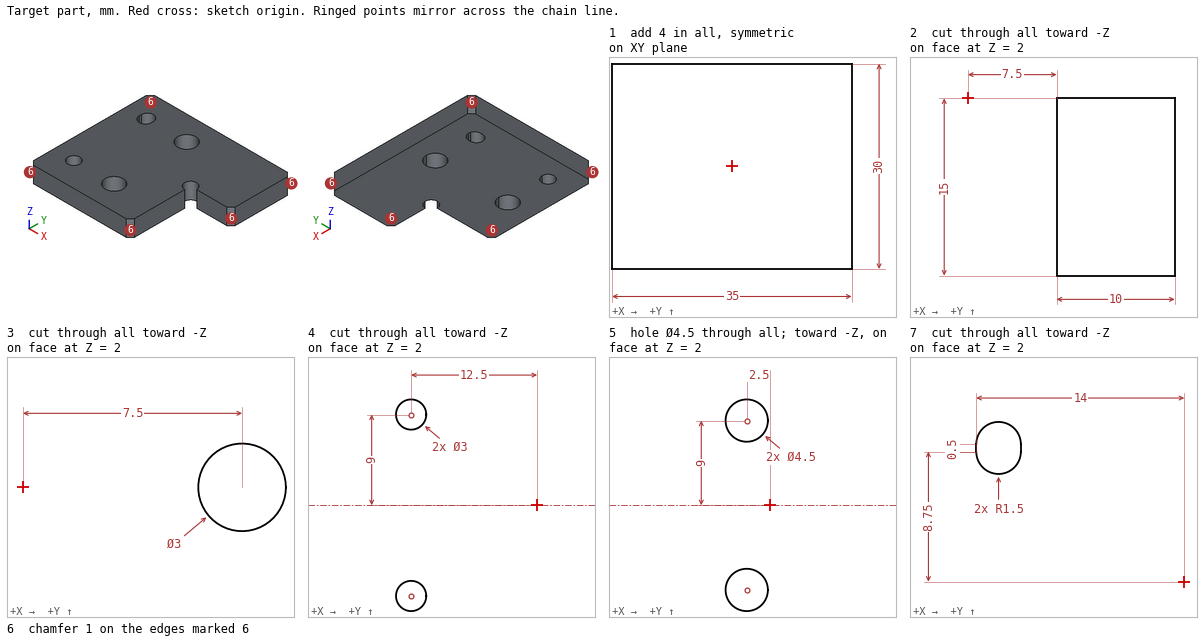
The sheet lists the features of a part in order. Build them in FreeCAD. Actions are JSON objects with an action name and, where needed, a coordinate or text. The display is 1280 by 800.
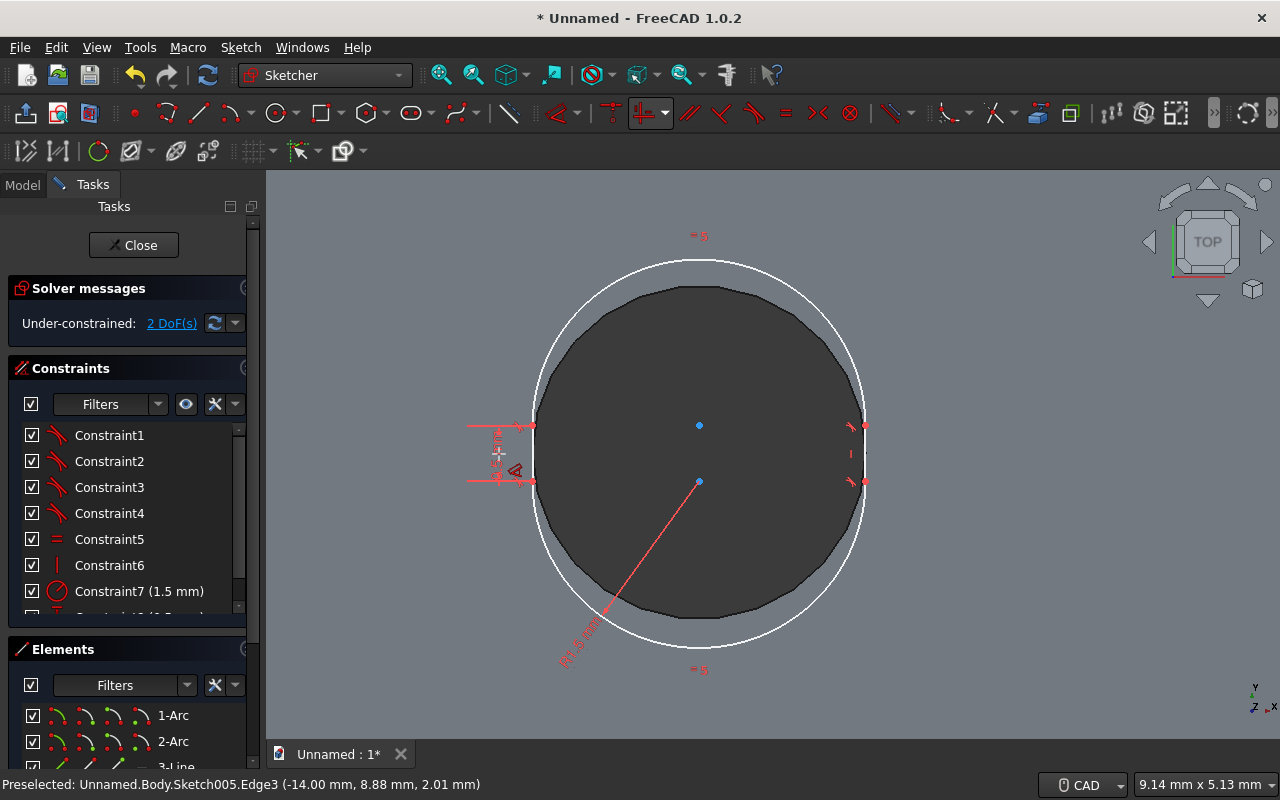
{"action": "left_click", "coordinate": [533, 481]}
{"action": "left_click", "coordinate": [824, 447]}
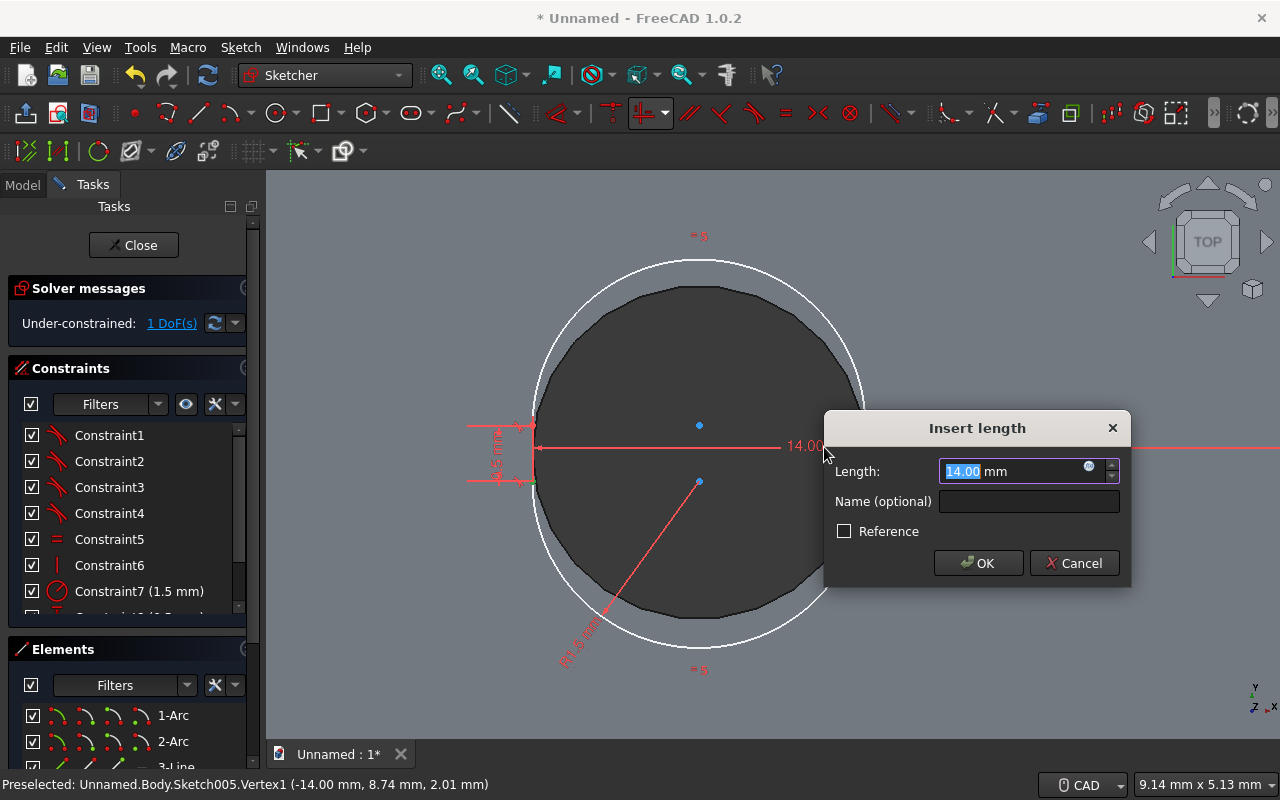
{"action": "type", "text": "14"}
{"action": "key", "text": "Return"}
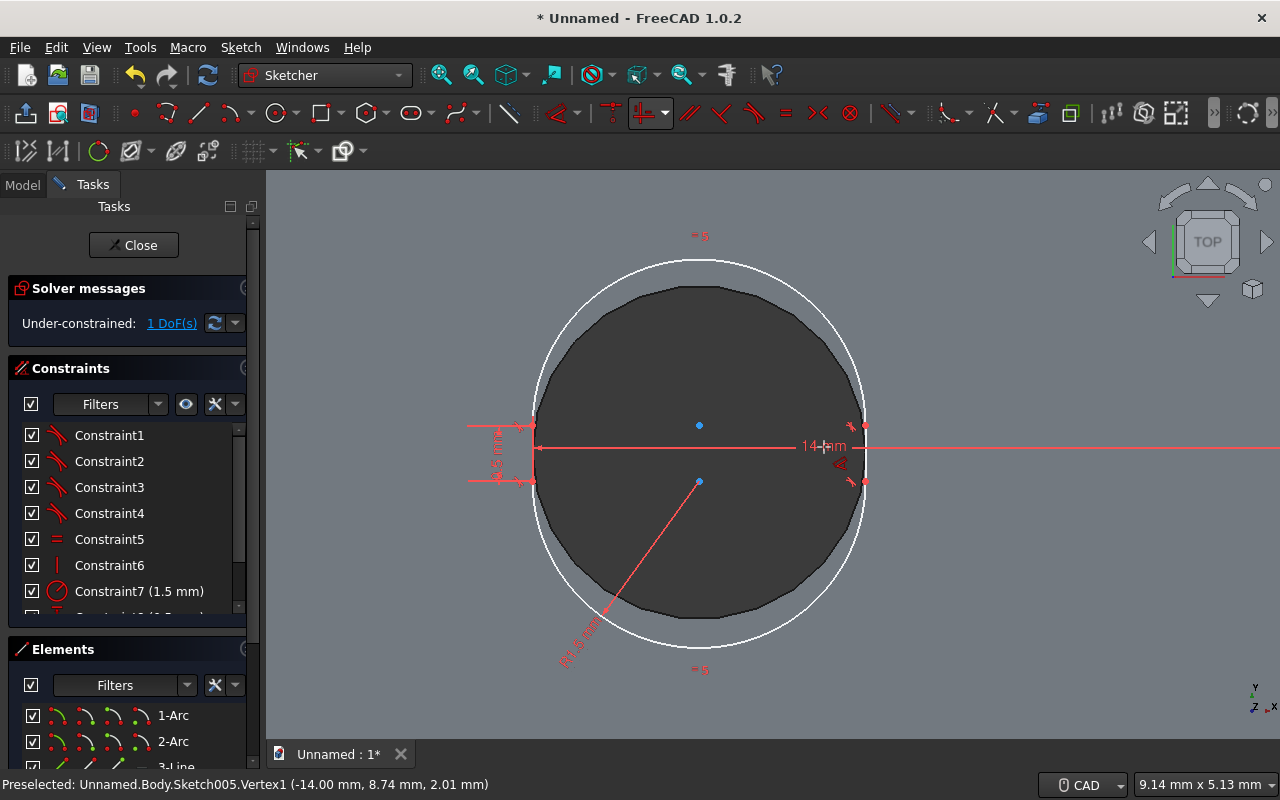
{"action": "left_click", "coordinate": [533, 481]}
{"action": "left_click", "coordinate": [499, 596]}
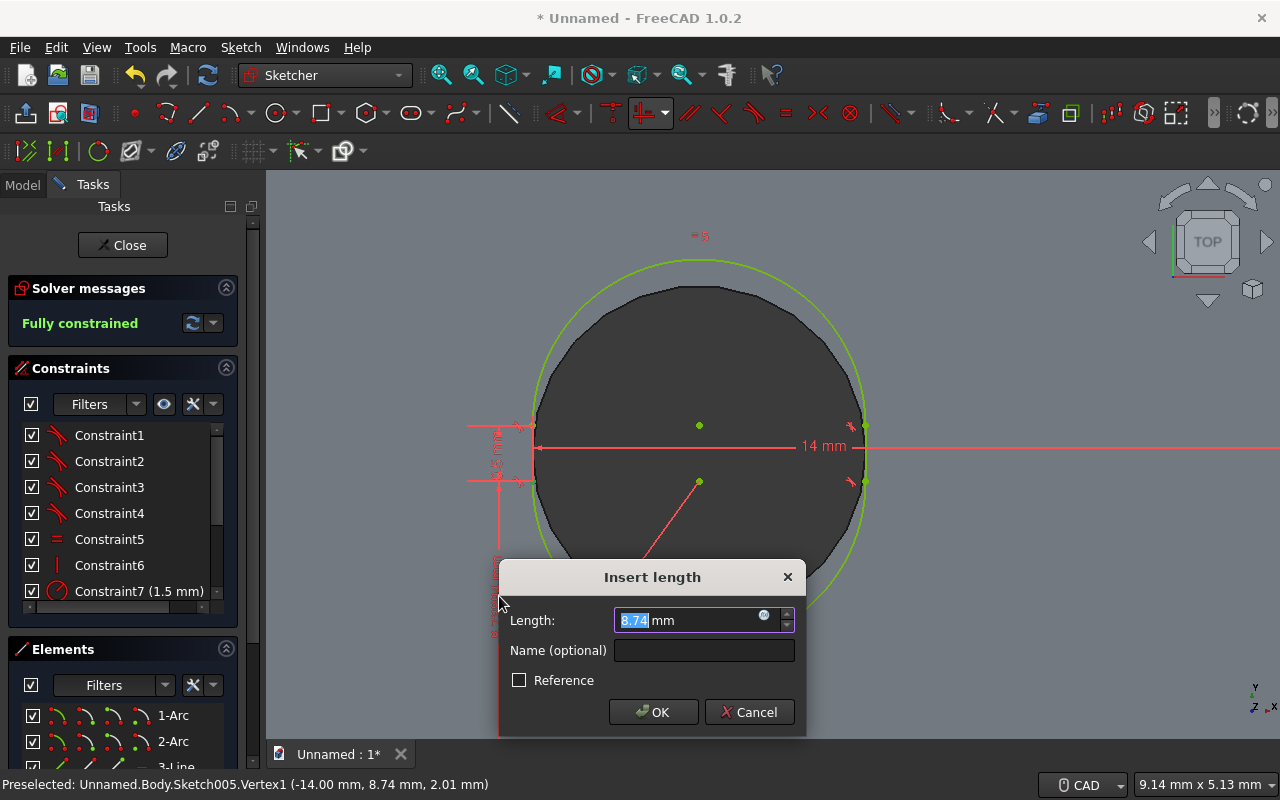
{"action": "type", "text": "8.75"}
{"action": "key", "text": "Return"}
{"action": "key", "text": "Escape"}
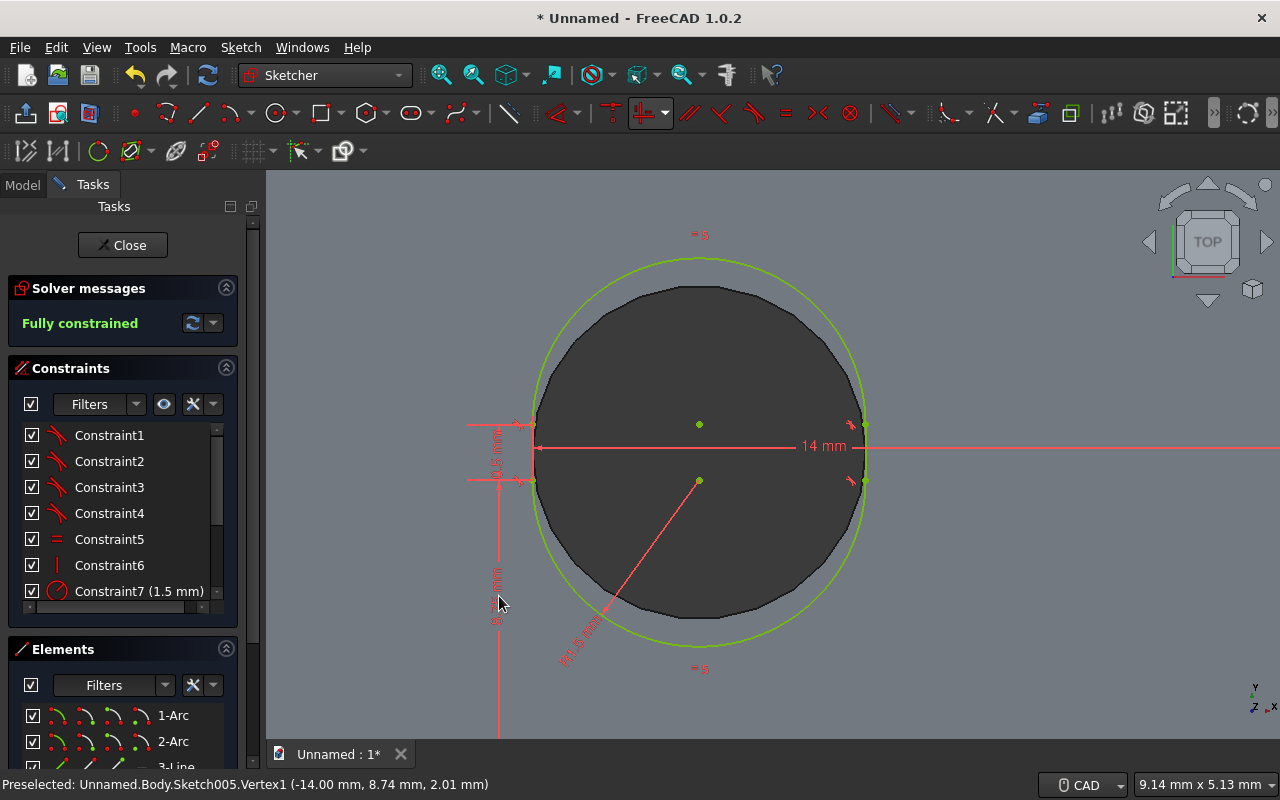
{"action": "left_click", "coordinate": [123, 245]}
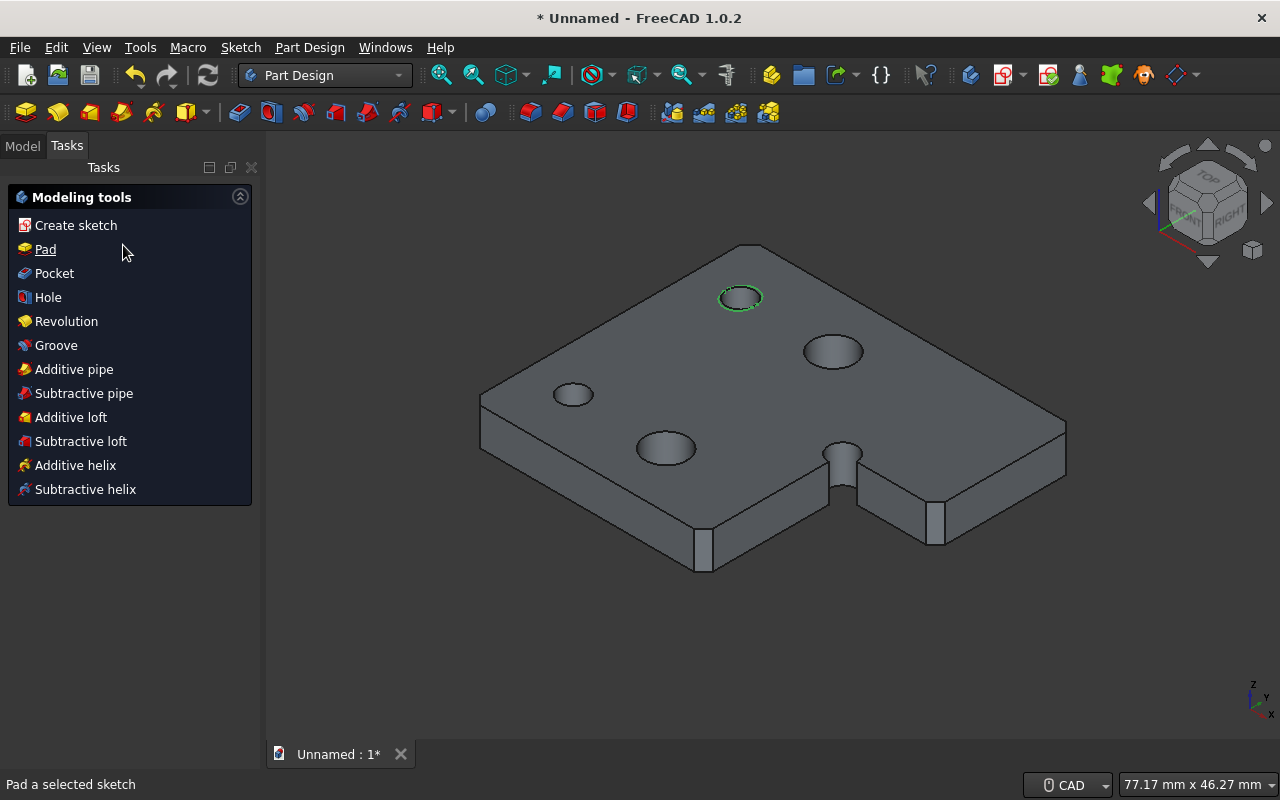
{"action": "left_click", "coordinate": [240, 112]}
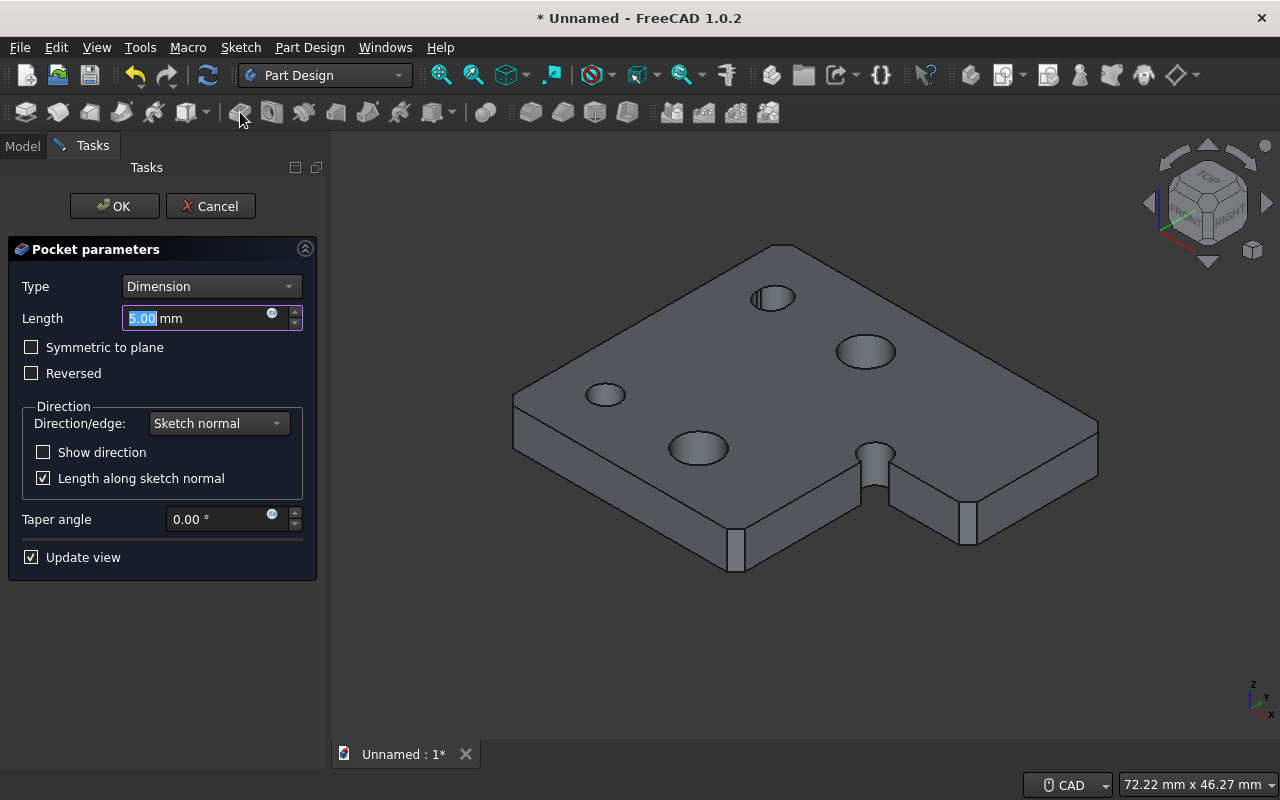
{"action": "left_click", "coordinate": [212, 286]}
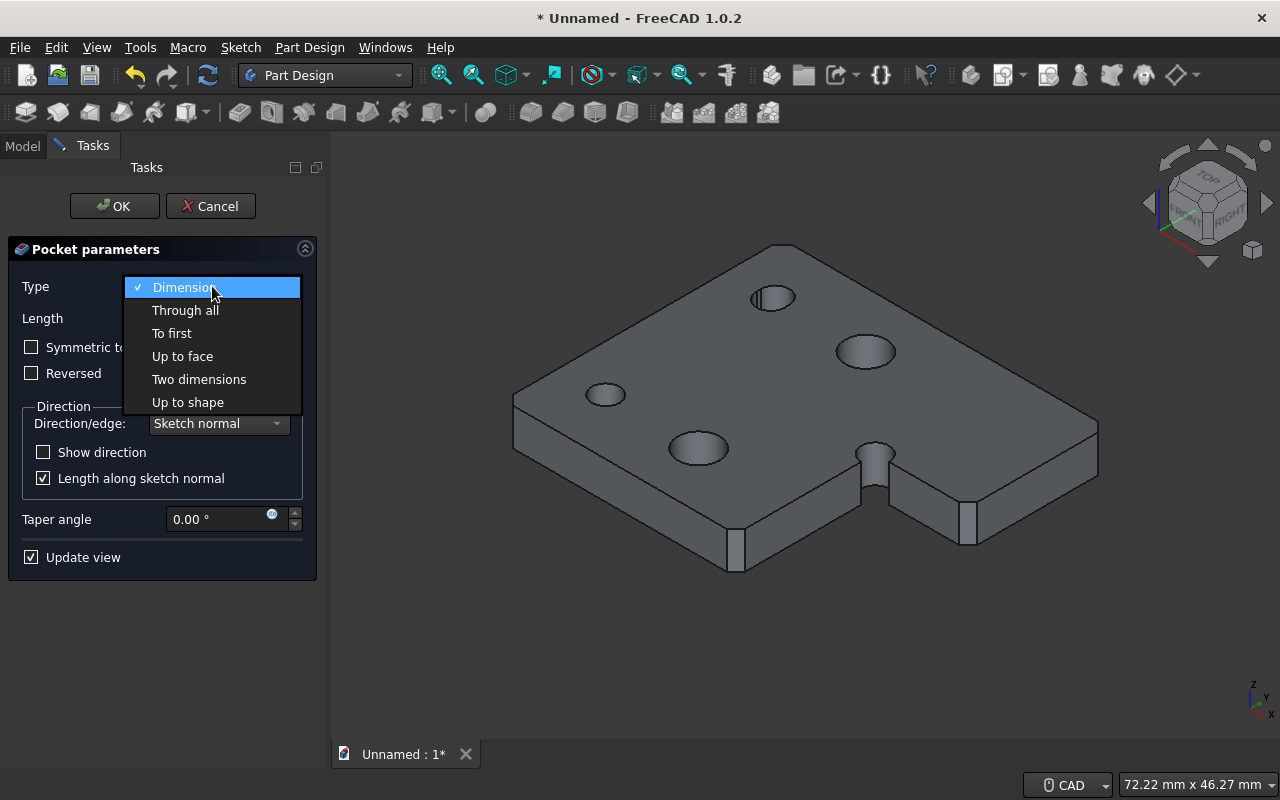
{"action": "left_click", "coordinate": [212, 310]}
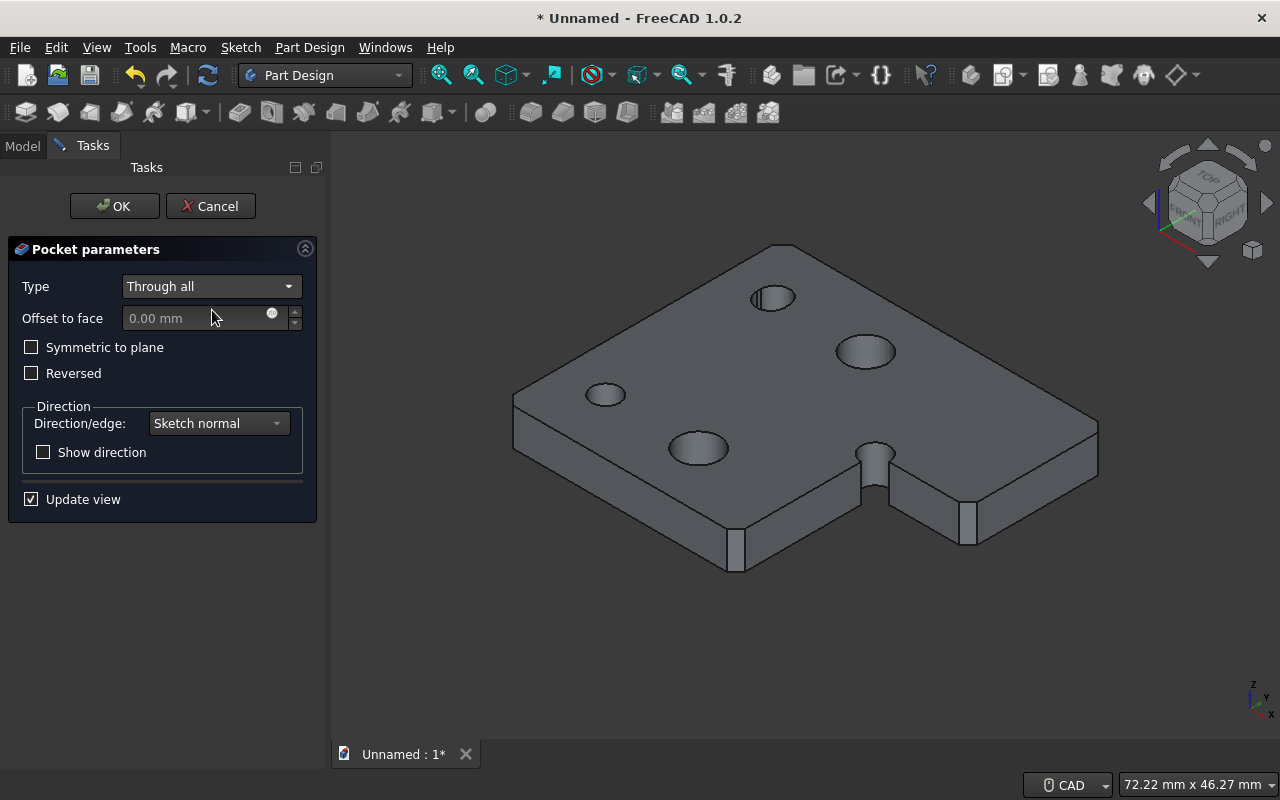
{"action": "left_click", "coordinate": [115, 206]}